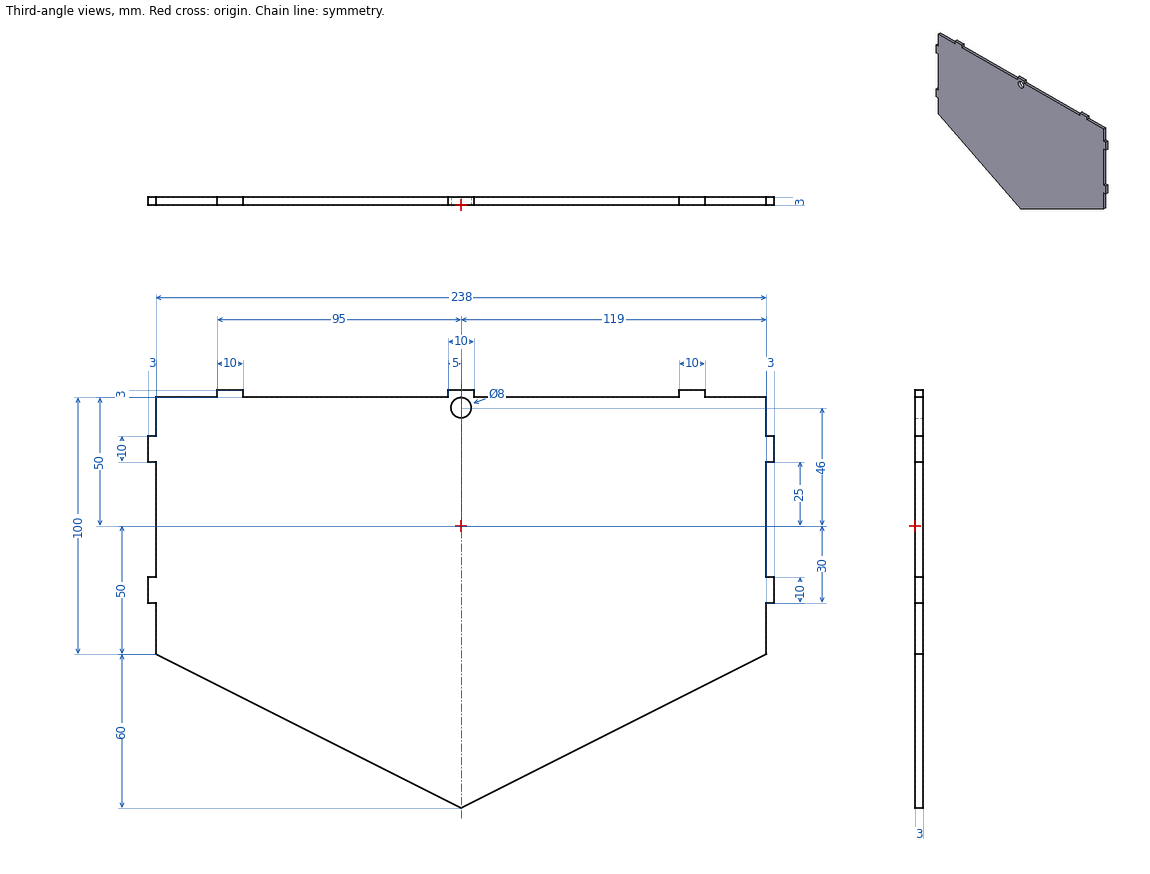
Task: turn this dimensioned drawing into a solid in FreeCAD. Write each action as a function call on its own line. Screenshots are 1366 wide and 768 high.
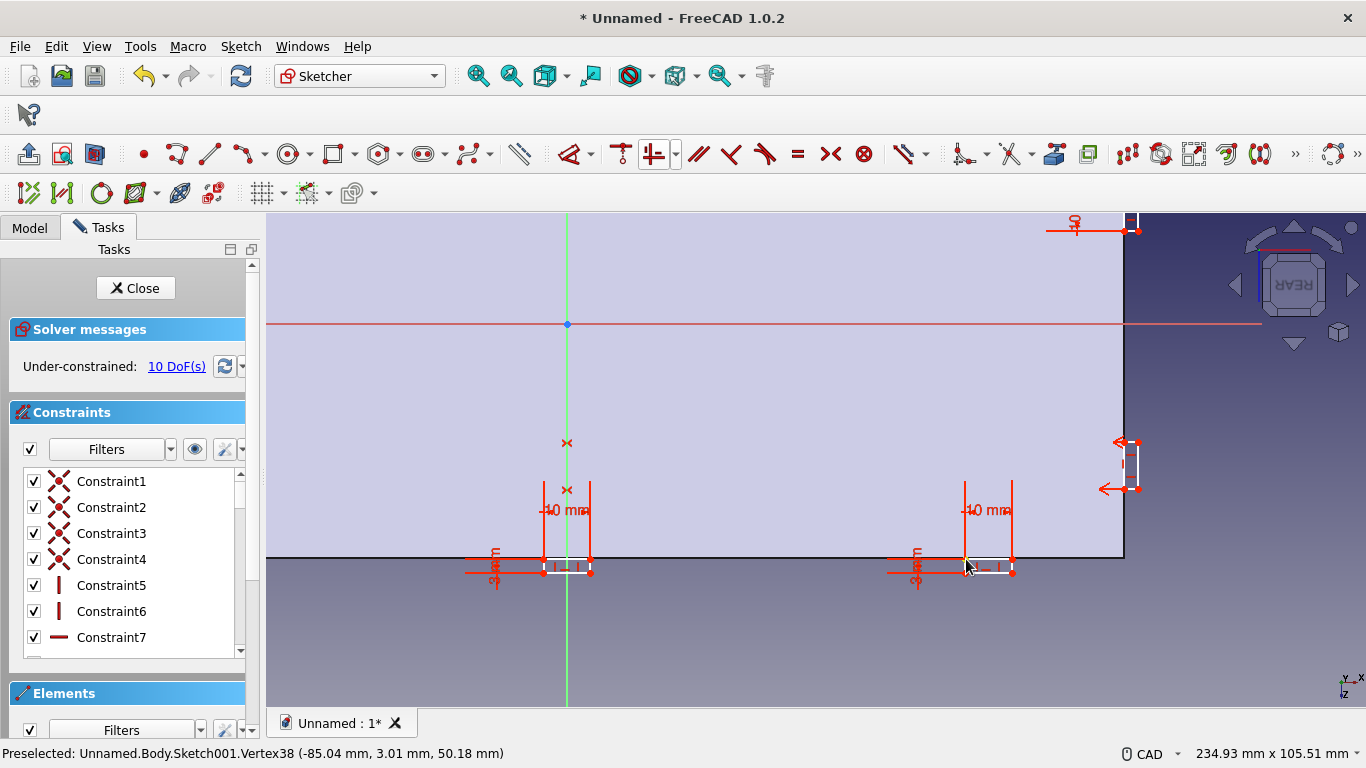
click(965, 559)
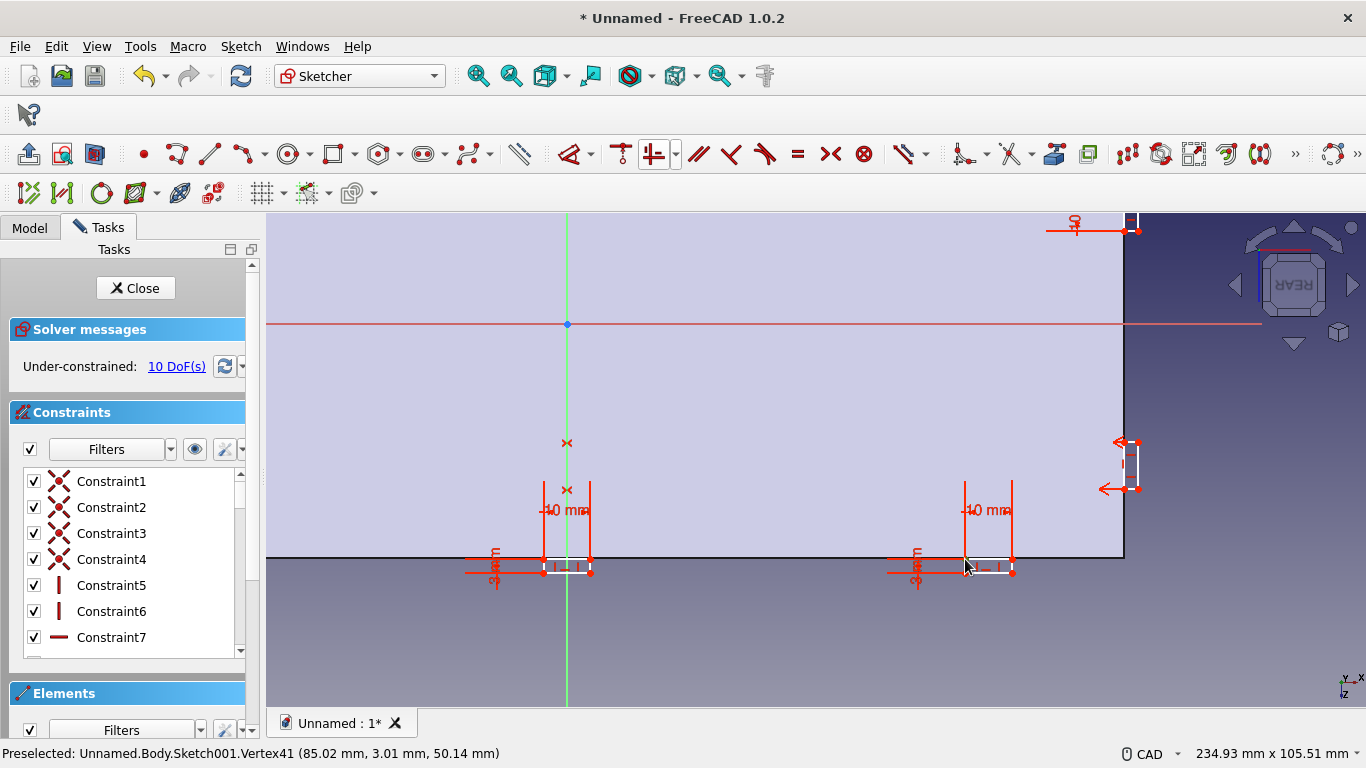
click(567, 648)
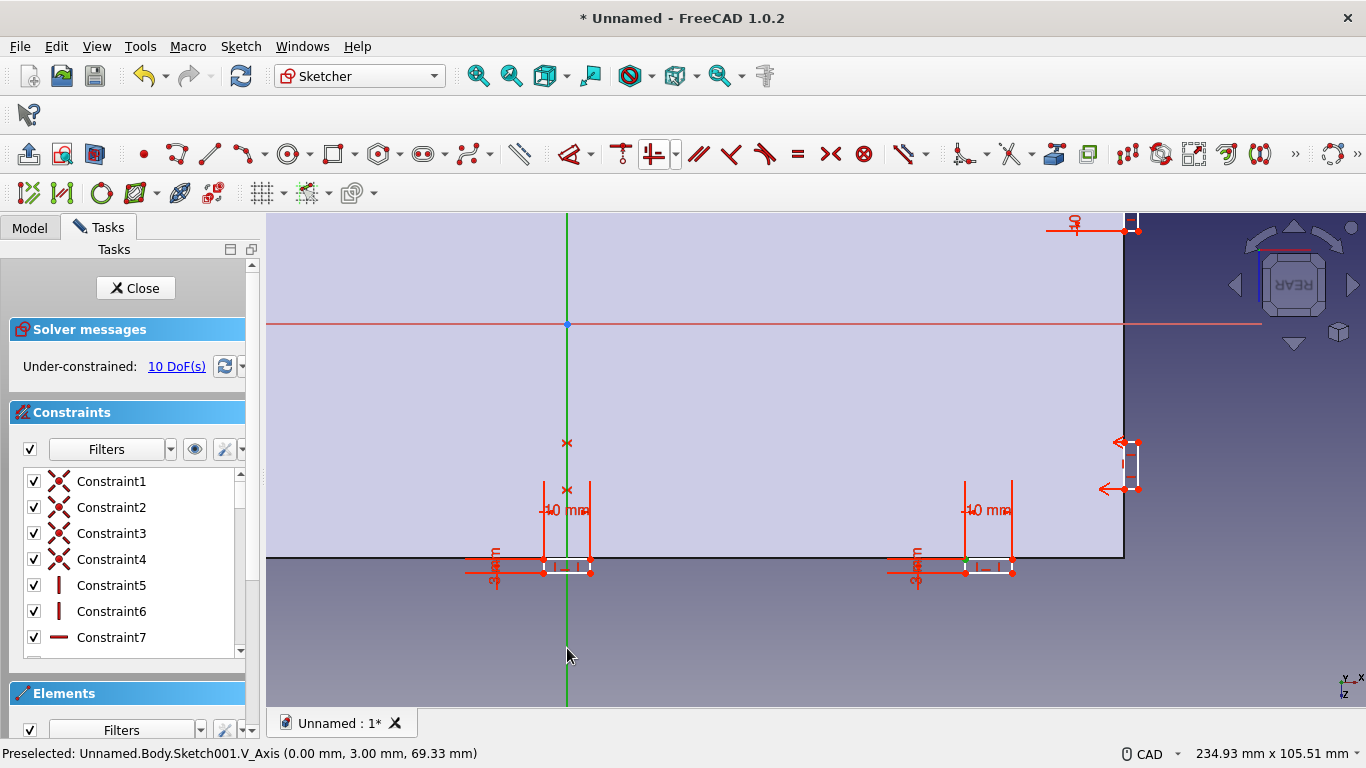
click(831, 154)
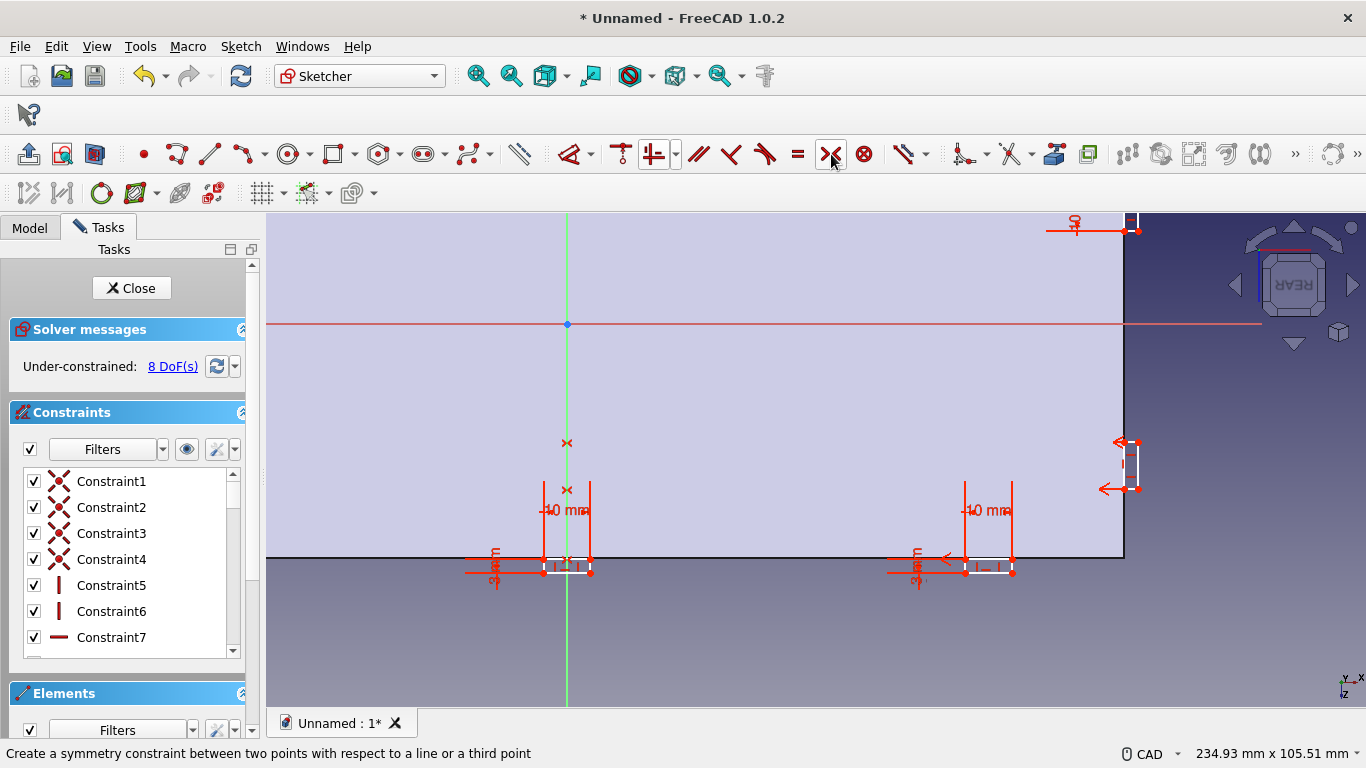
click(568, 154)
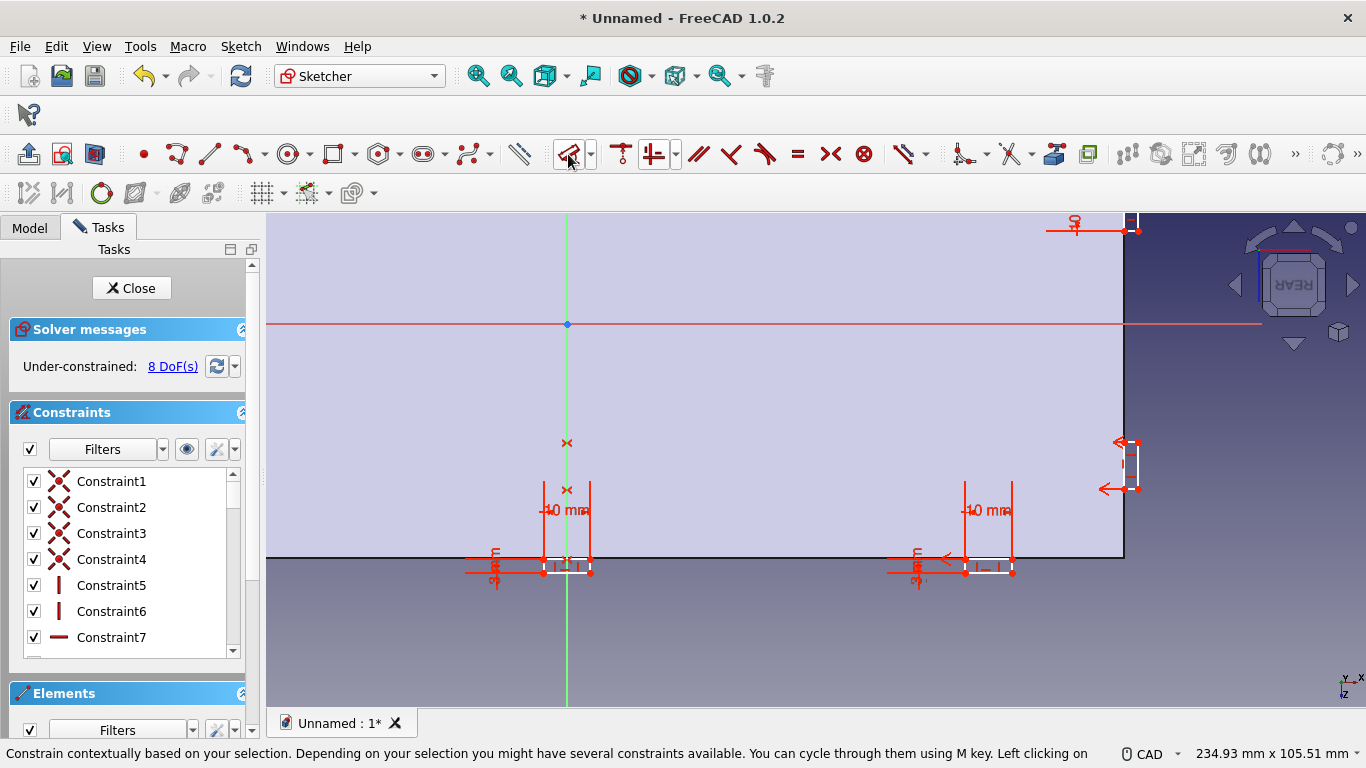
scroll(544, 559, up, 3)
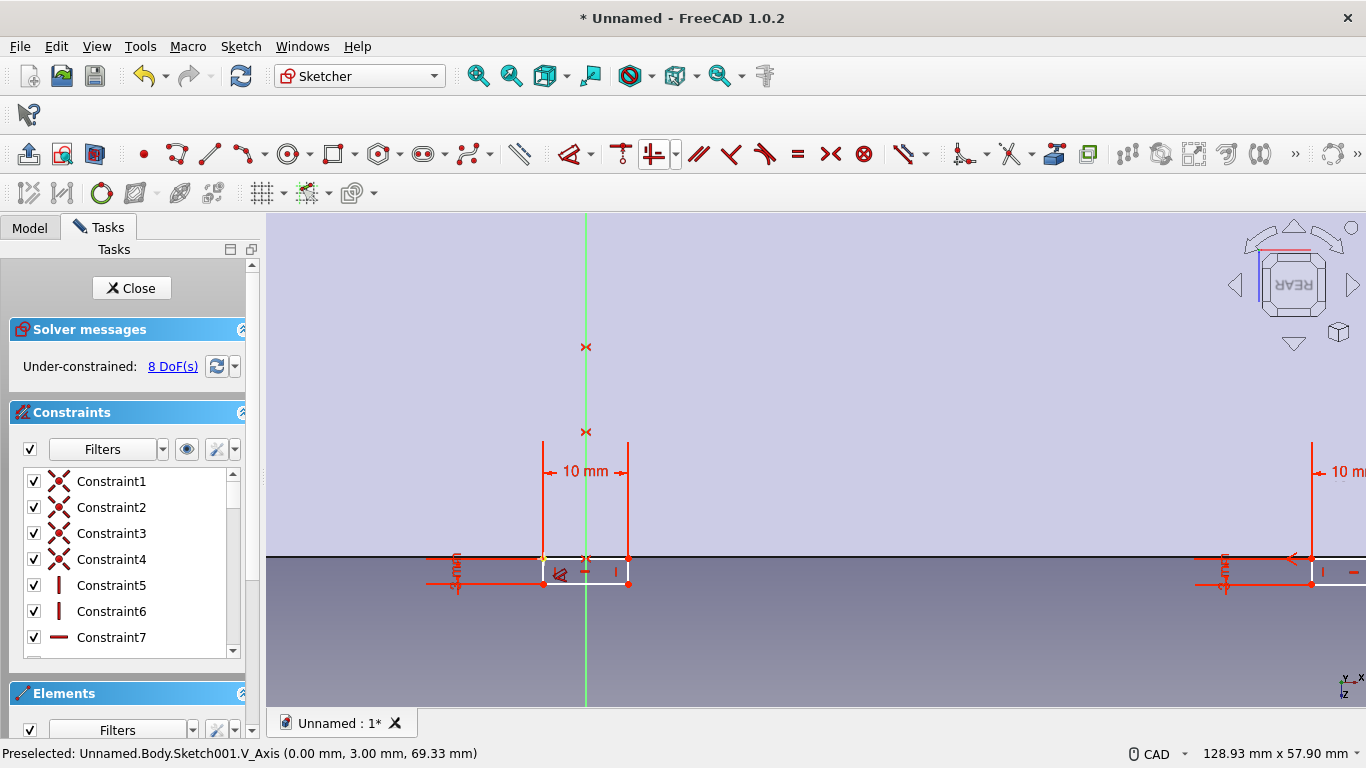
click(543, 559)
click(565, 617)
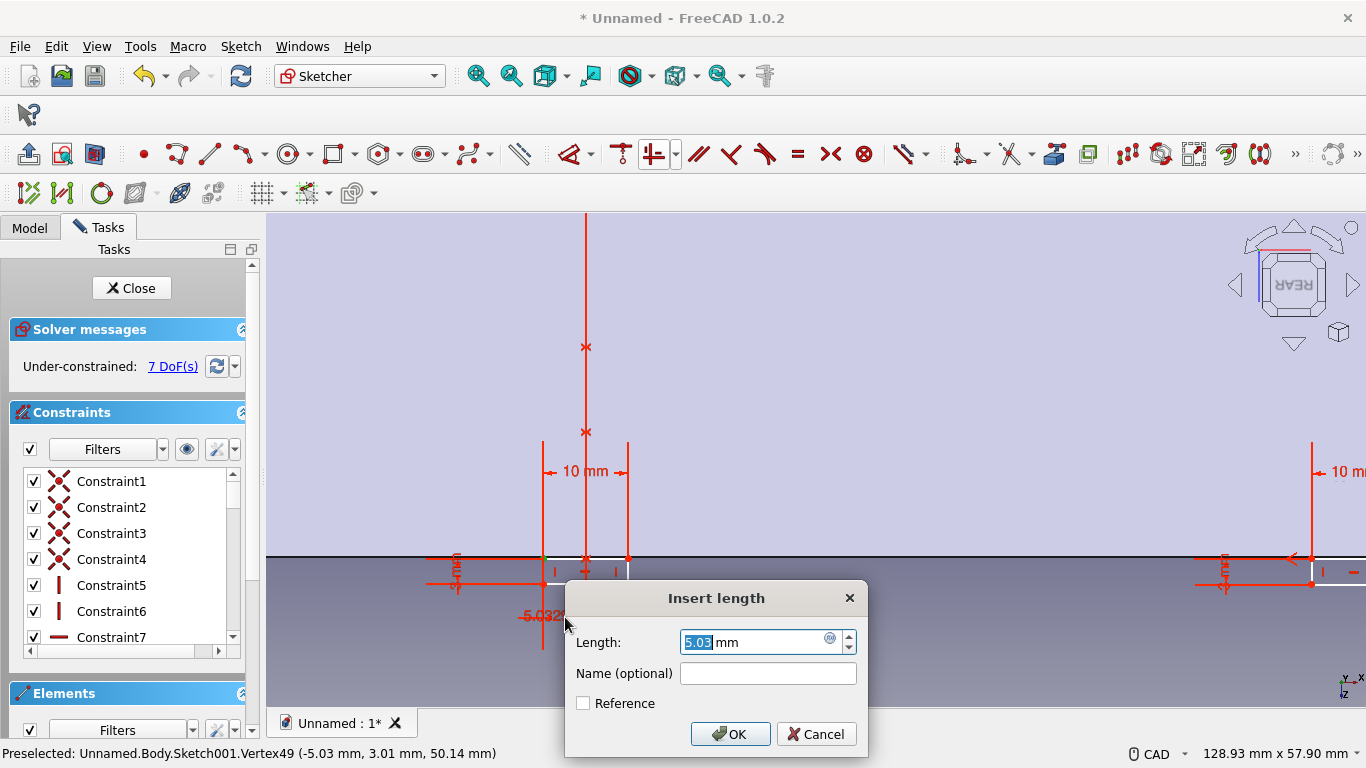
text(5)
key(Return)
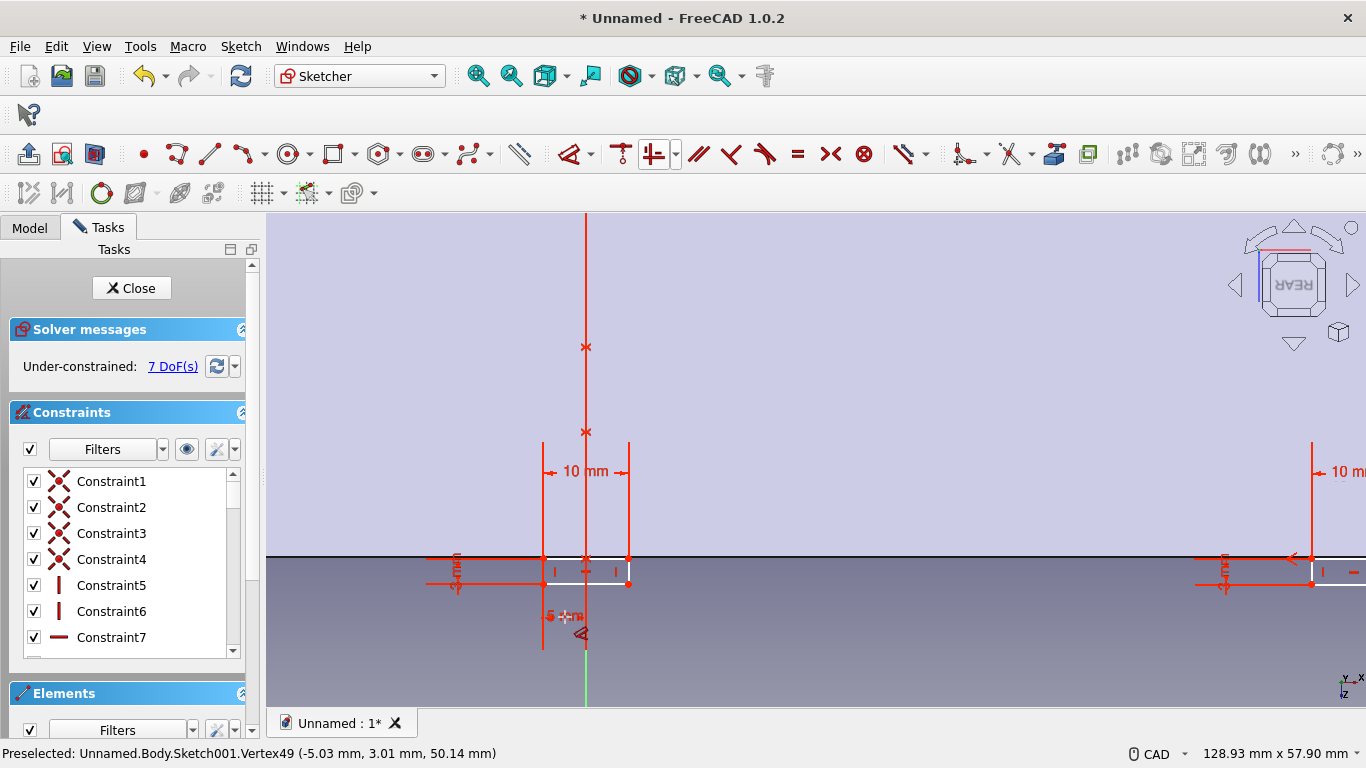
scroll(817, 560, down, 6)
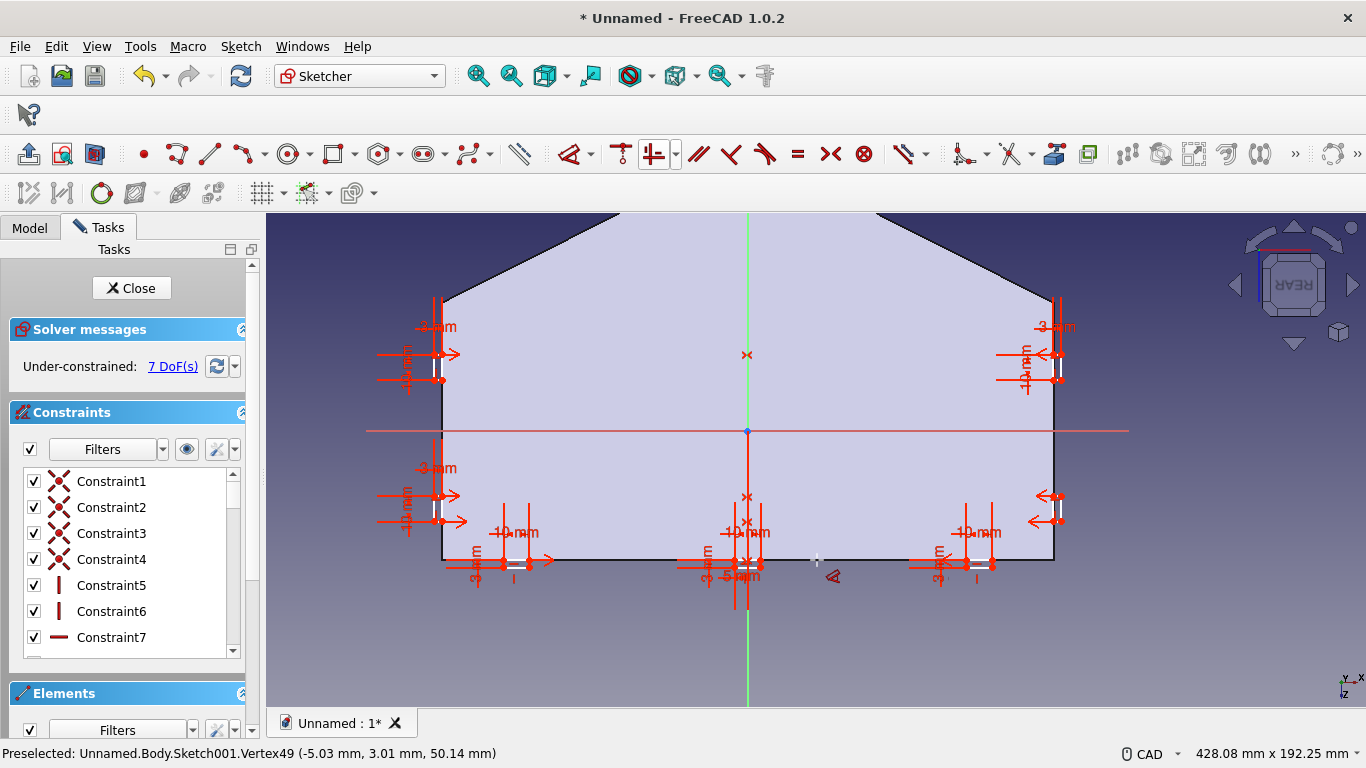
scroll(1053, 355, up, 3)